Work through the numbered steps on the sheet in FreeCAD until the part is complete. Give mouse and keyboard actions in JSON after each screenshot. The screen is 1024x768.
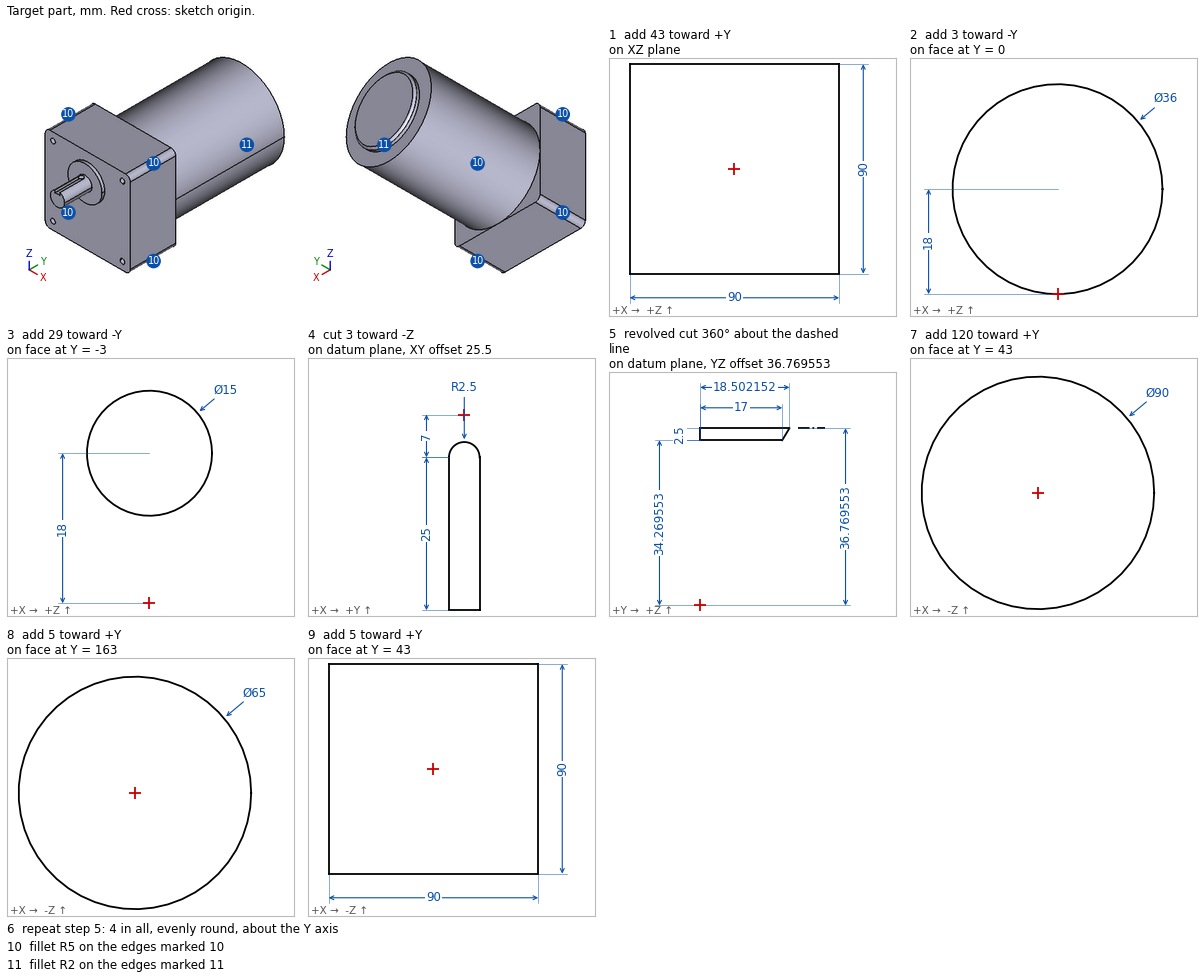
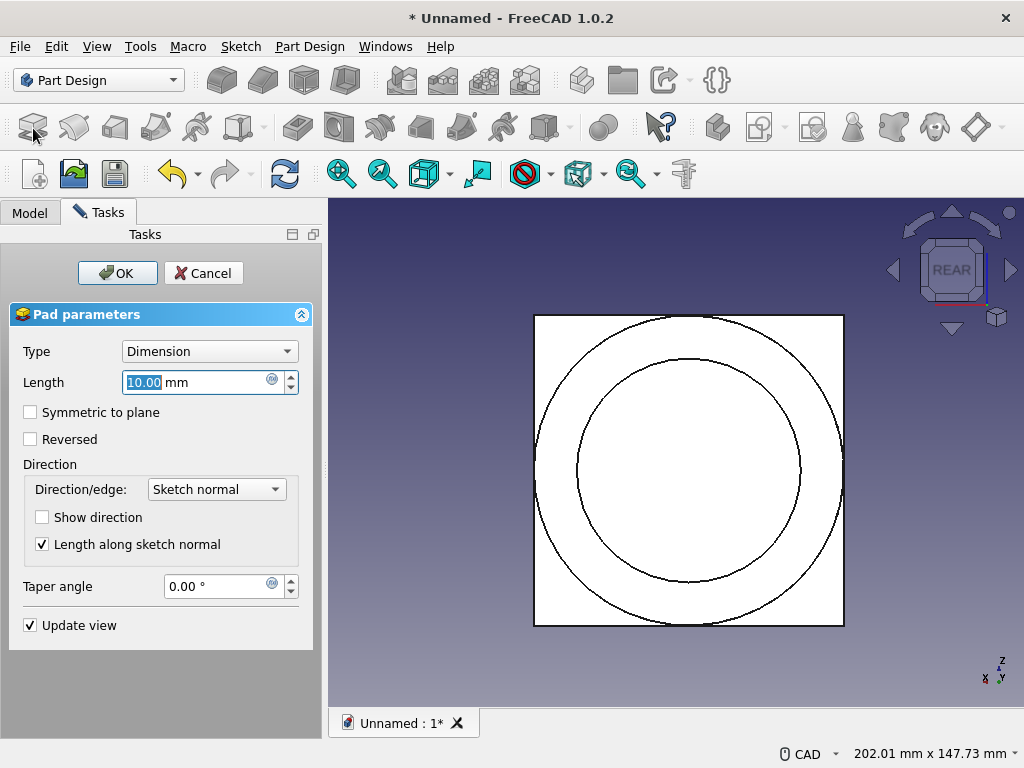
{"action": "type", "text": "5"}
{"action": "key", "text": "Tab"}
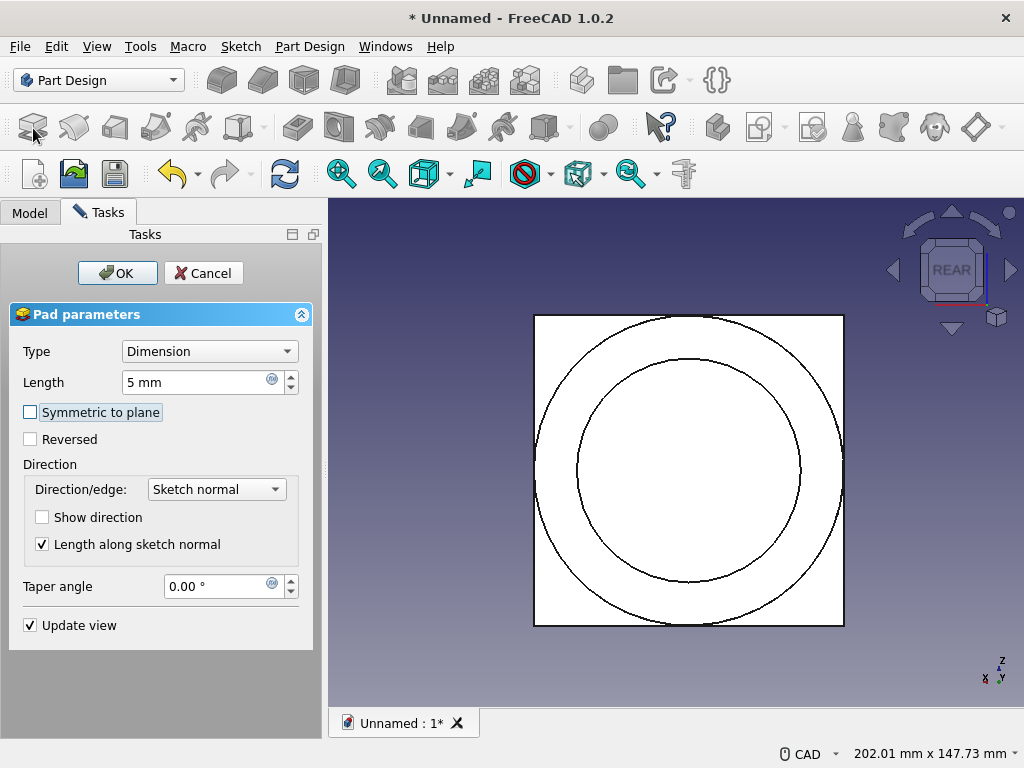
{"action": "left_click", "coordinate": [118, 273]}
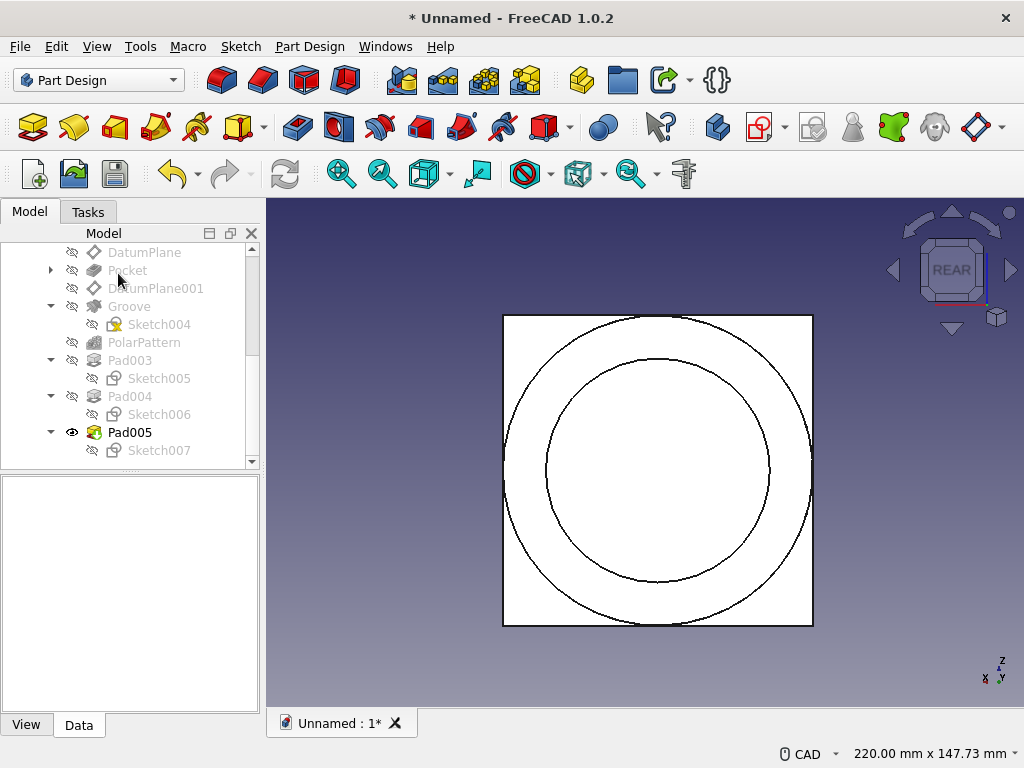
{"action": "key", "text": "0"}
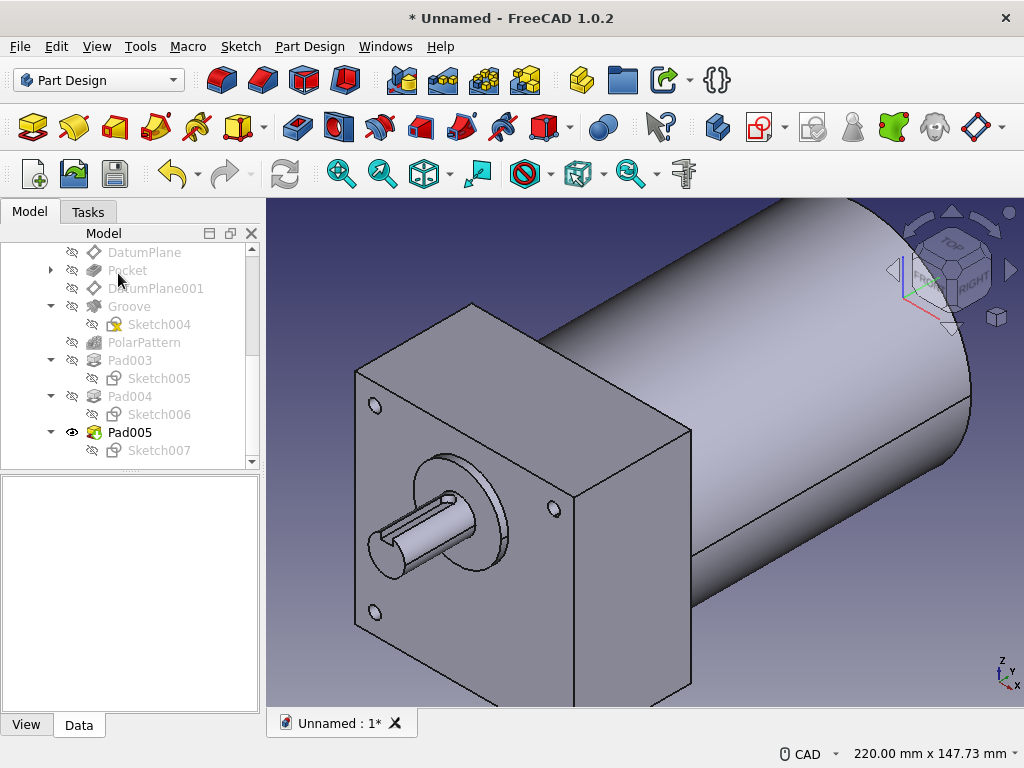
{"action": "left_click", "coordinate": [342, 174]}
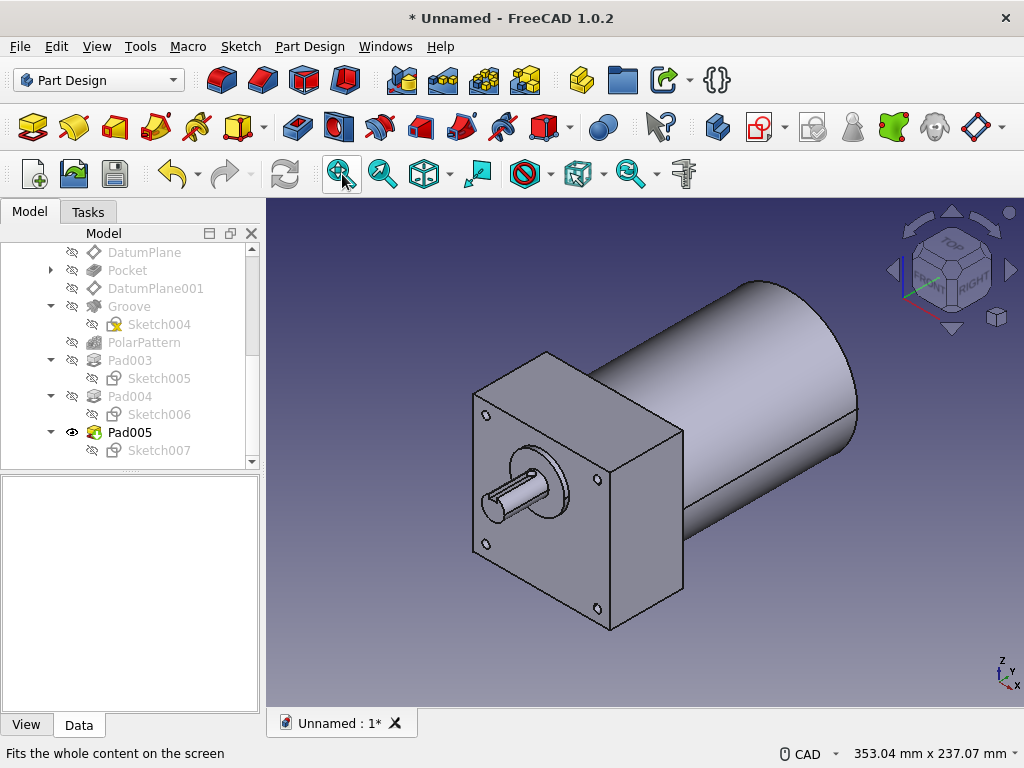
{"action": "left_click", "coordinate": [647, 451]}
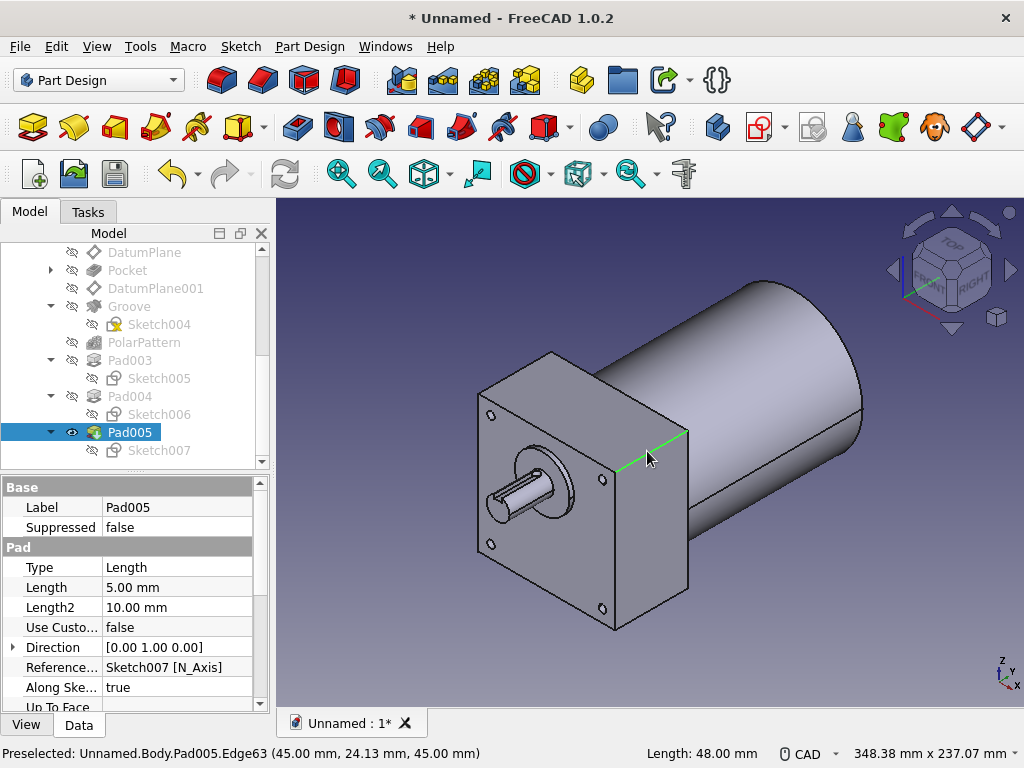
{"action": "key", "text": "2"}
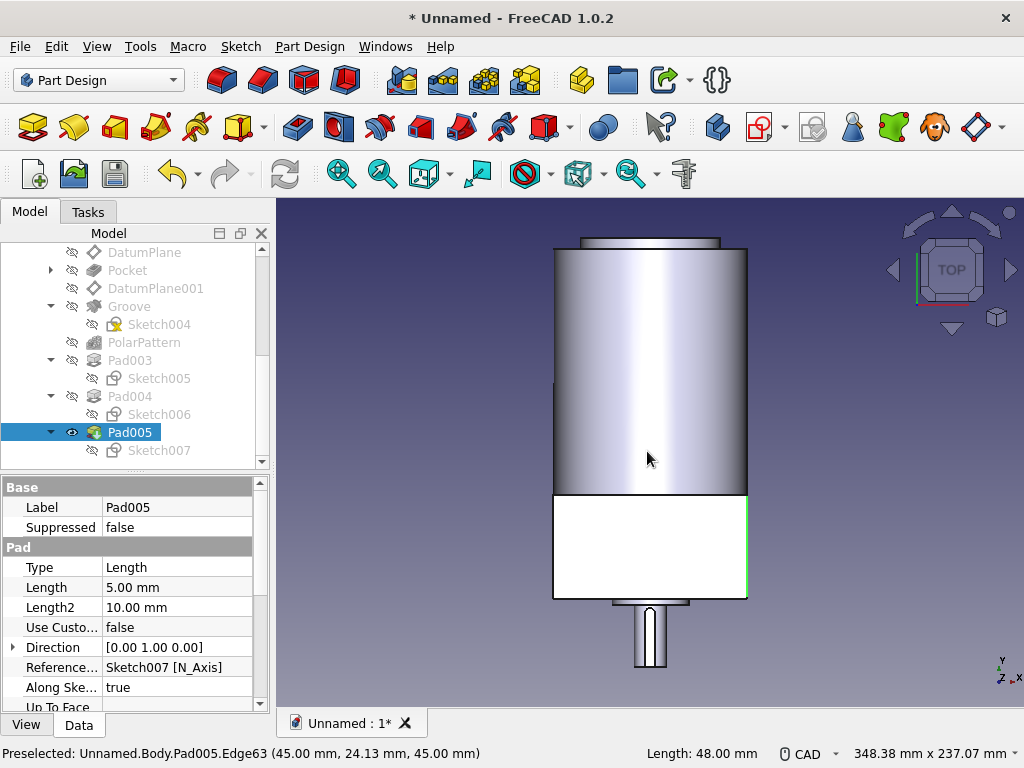
{"action": "left_click", "coordinate": [553, 546], "text": "ctrl"}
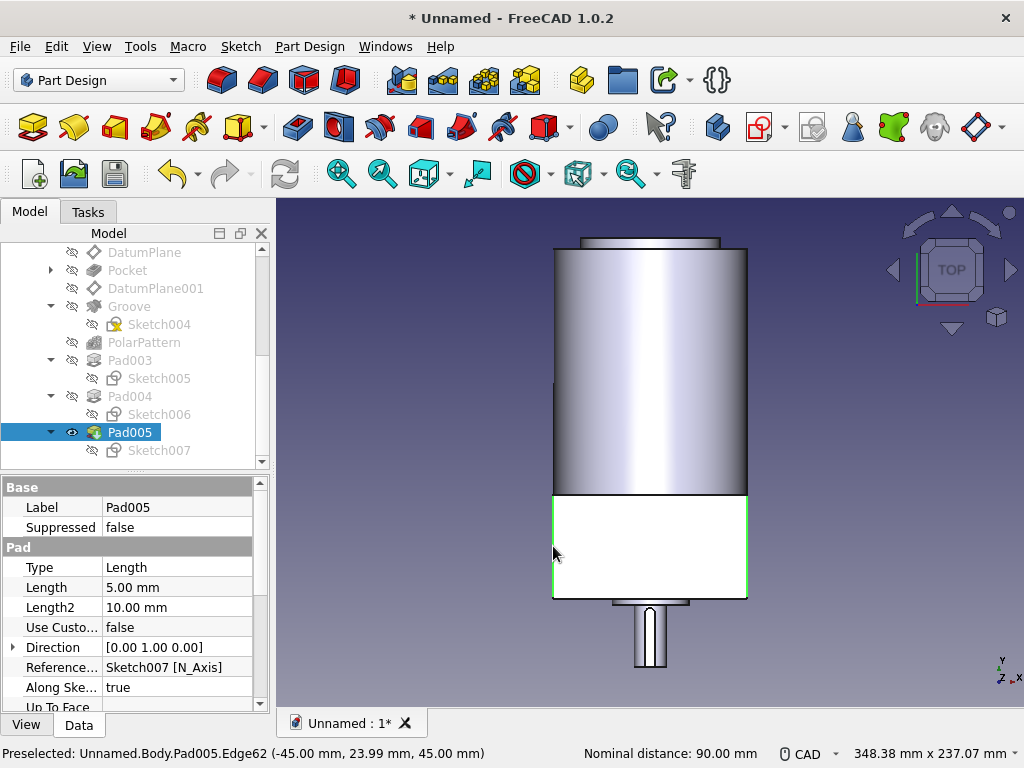
{"action": "key", "text": "1"}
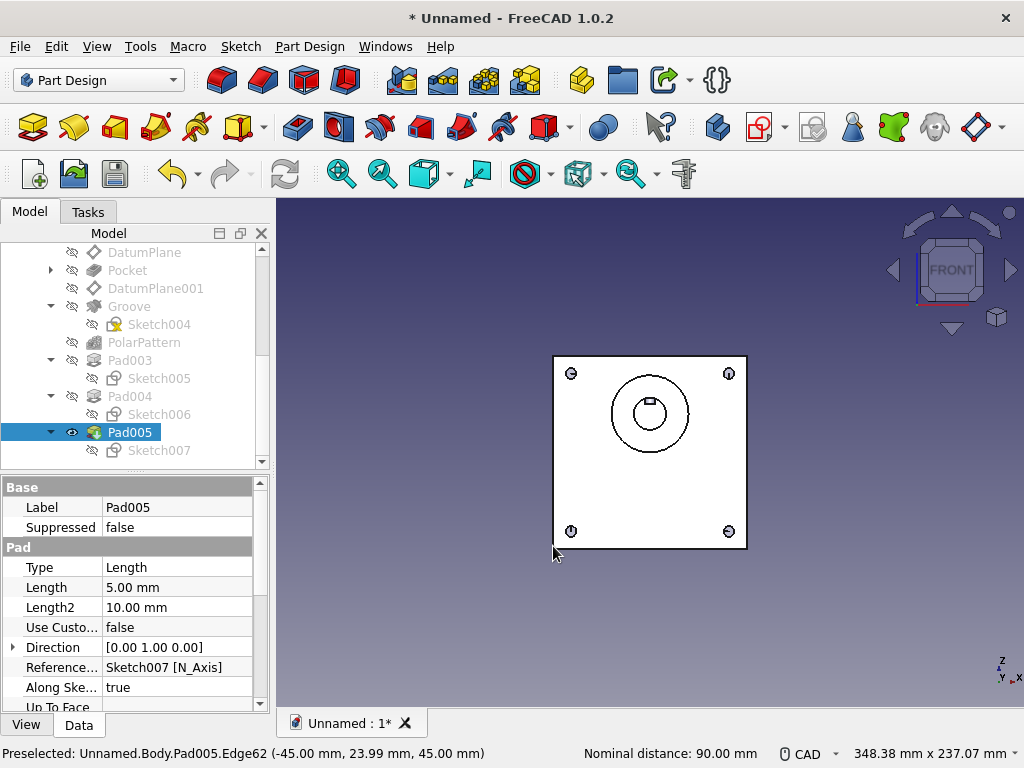
{"action": "key", "text": "v f"}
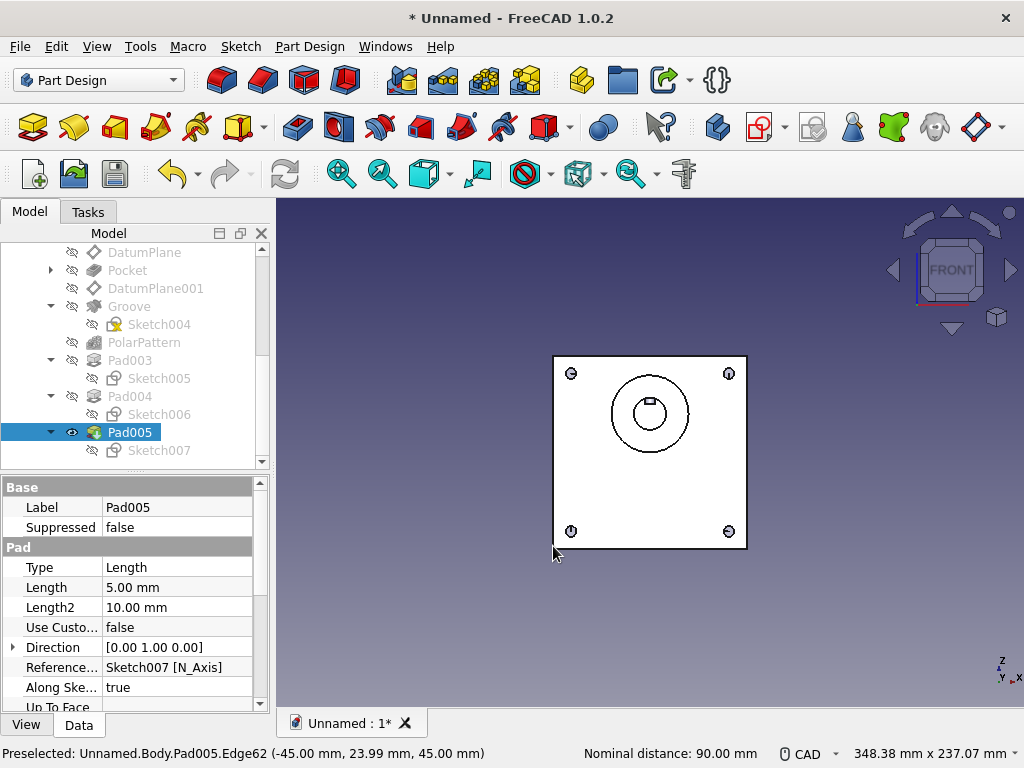
{"action": "key", "text": "3"}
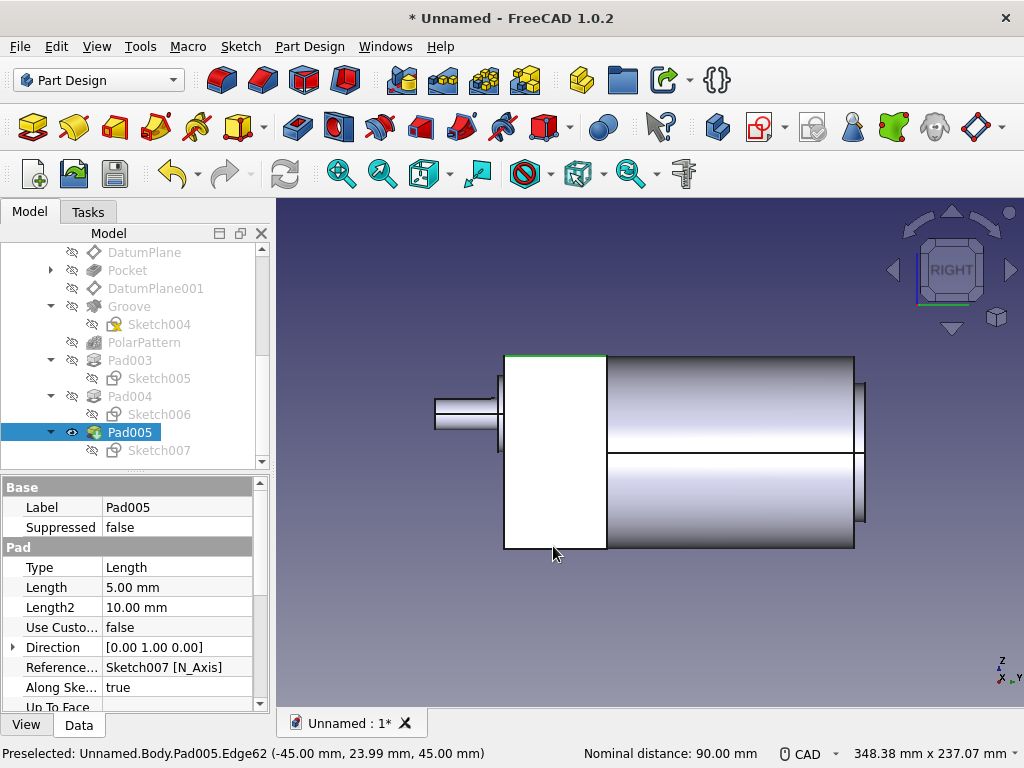
{"action": "left_click", "coordinate": [556, 548], "text": "ctrl"}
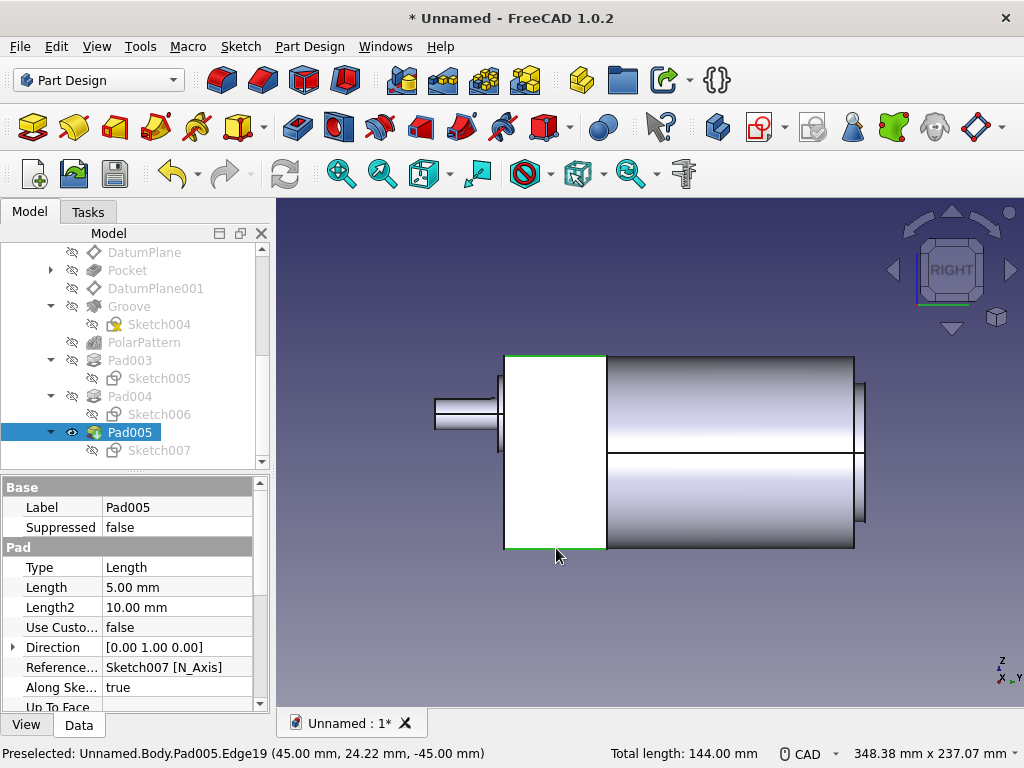
{"action": "key", "text": "5"}